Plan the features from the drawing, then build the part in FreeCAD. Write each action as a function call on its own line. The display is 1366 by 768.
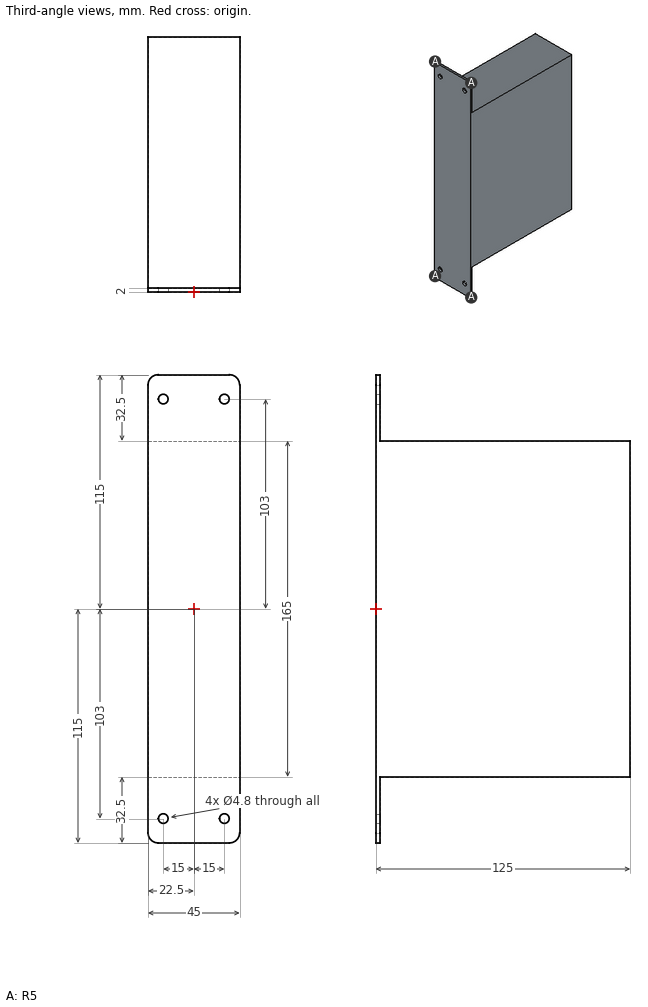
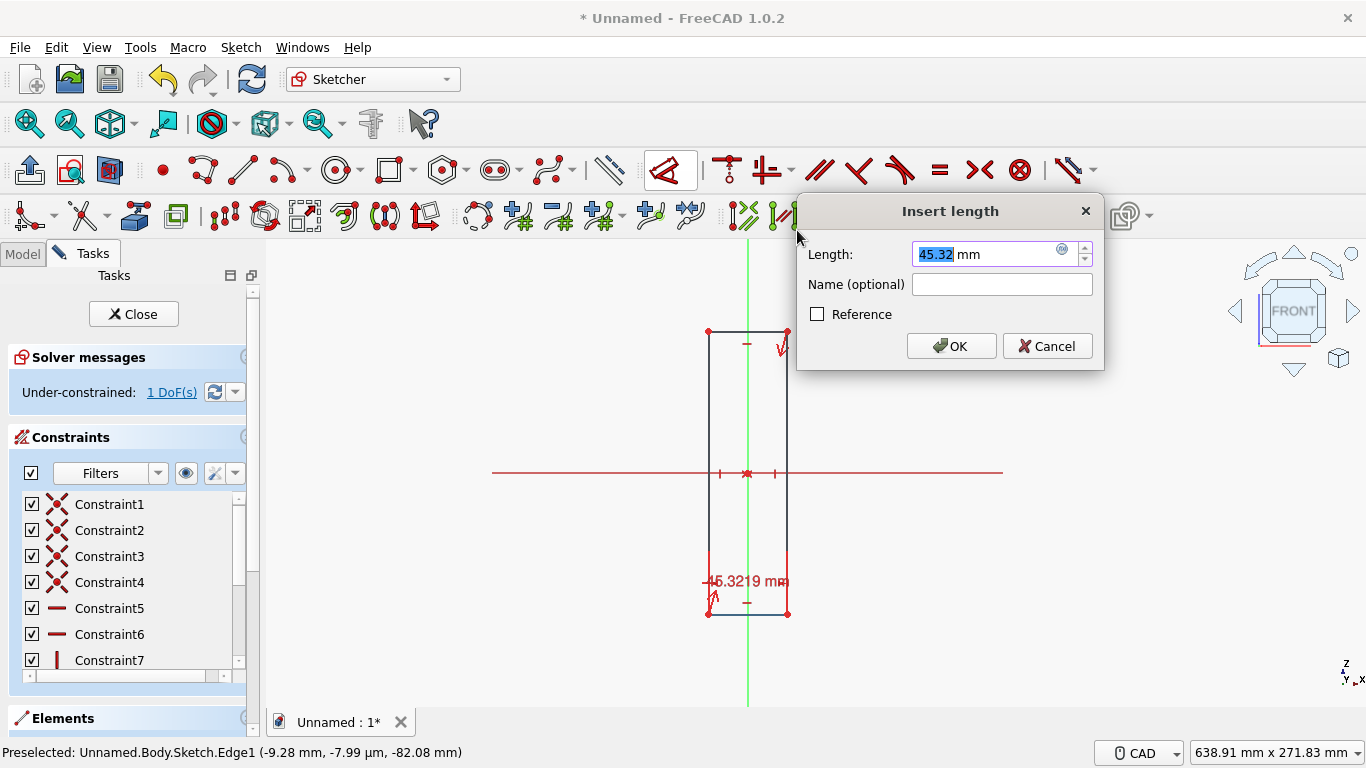
text(45)
key(Return)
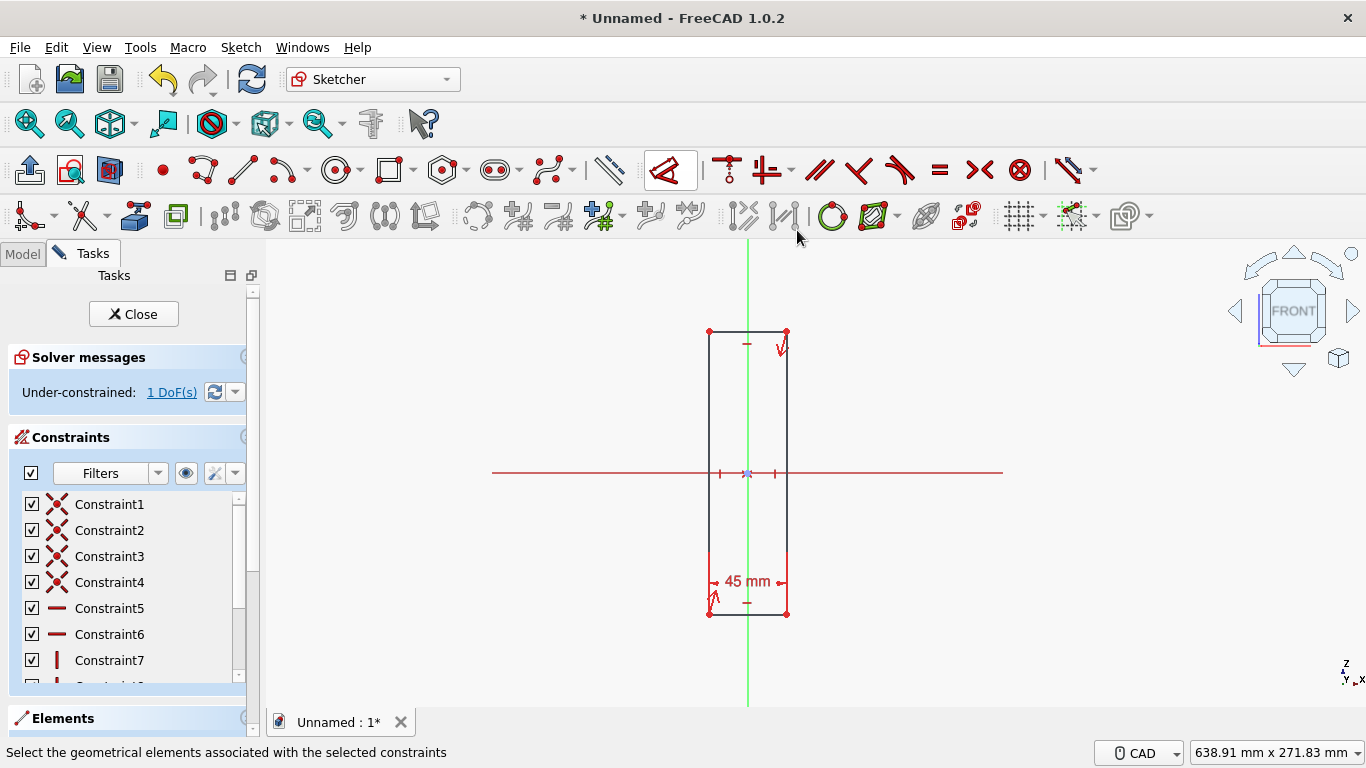
click(787, 530)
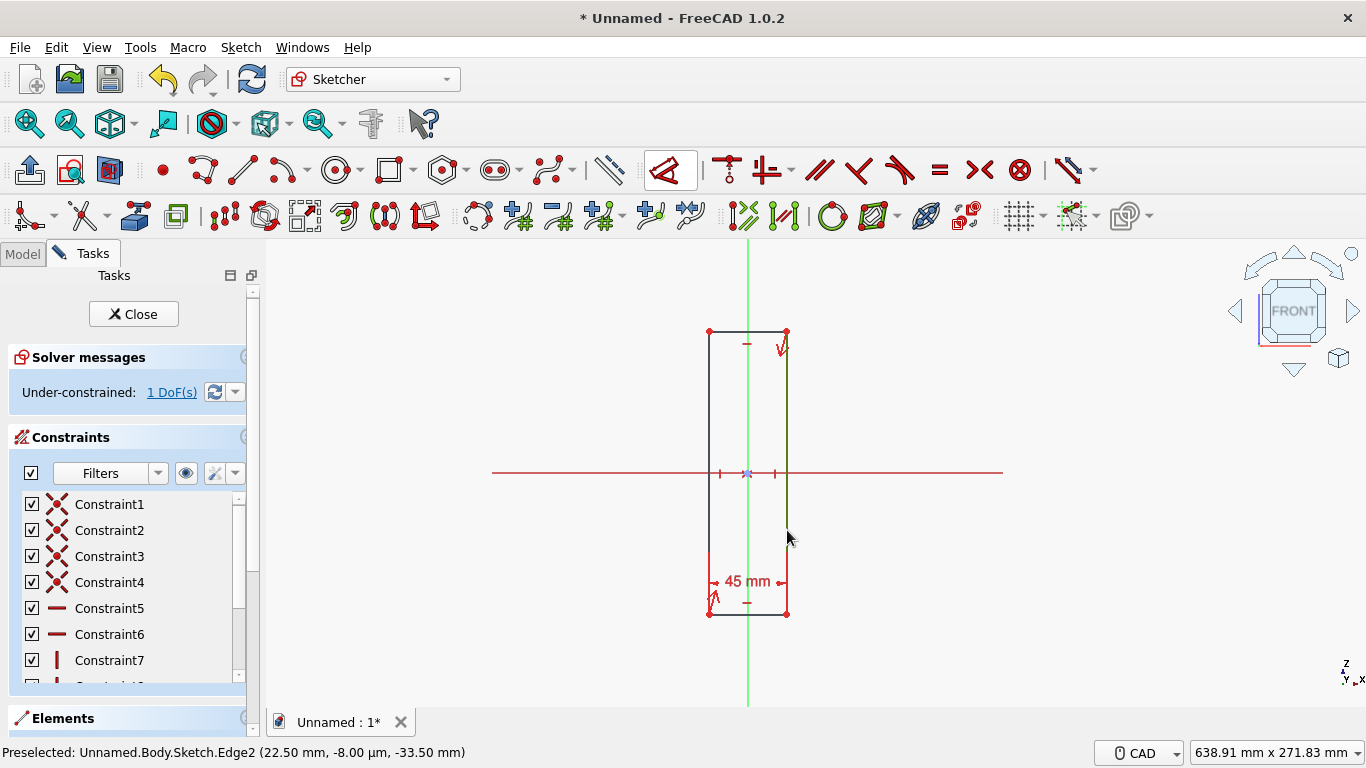
key(i)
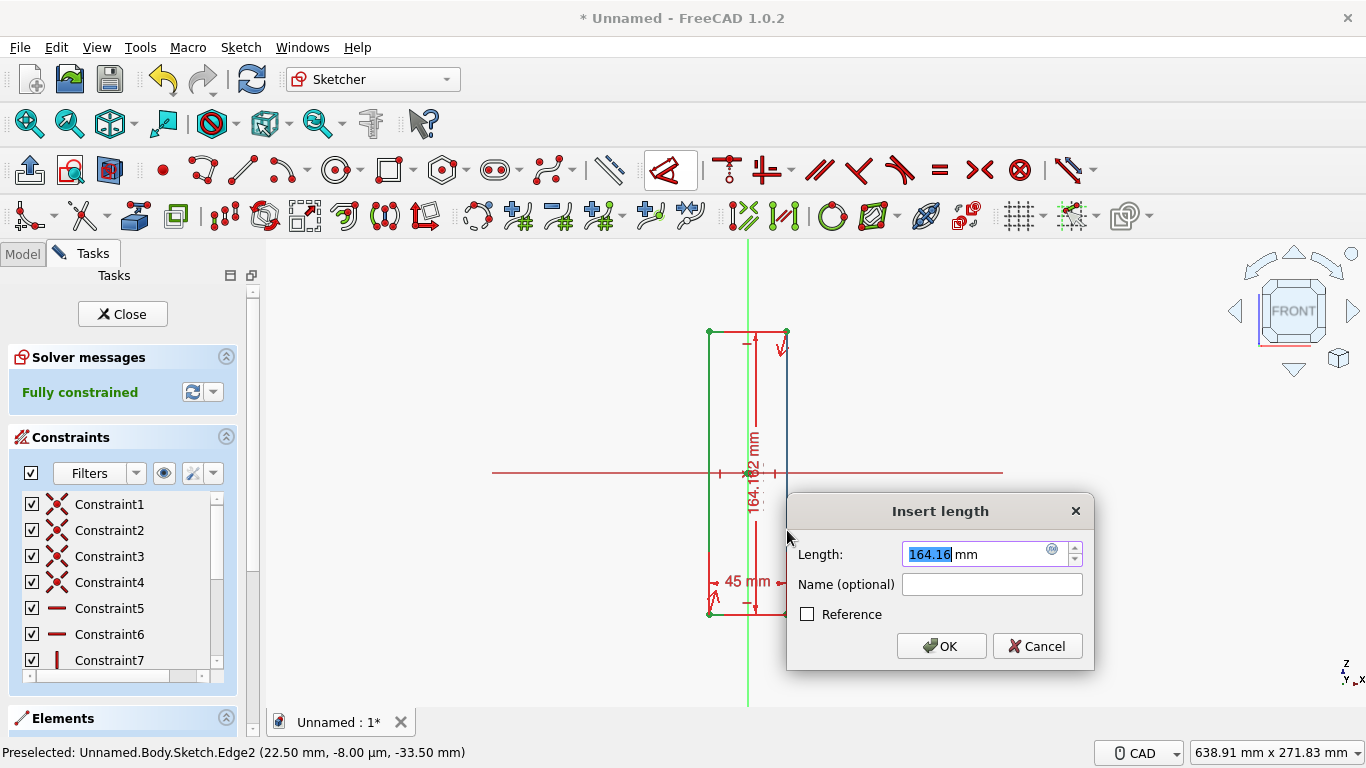
text(165)
key(Return)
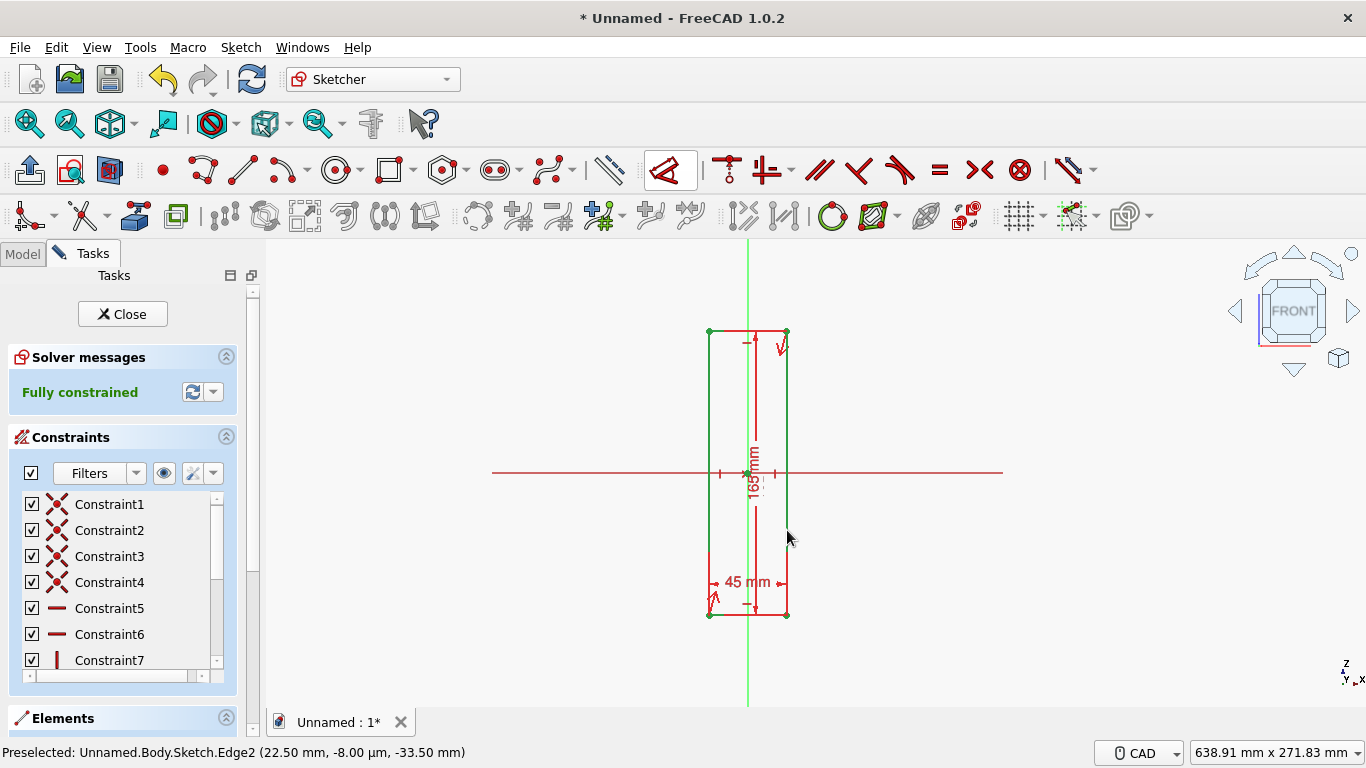
click(123, 314)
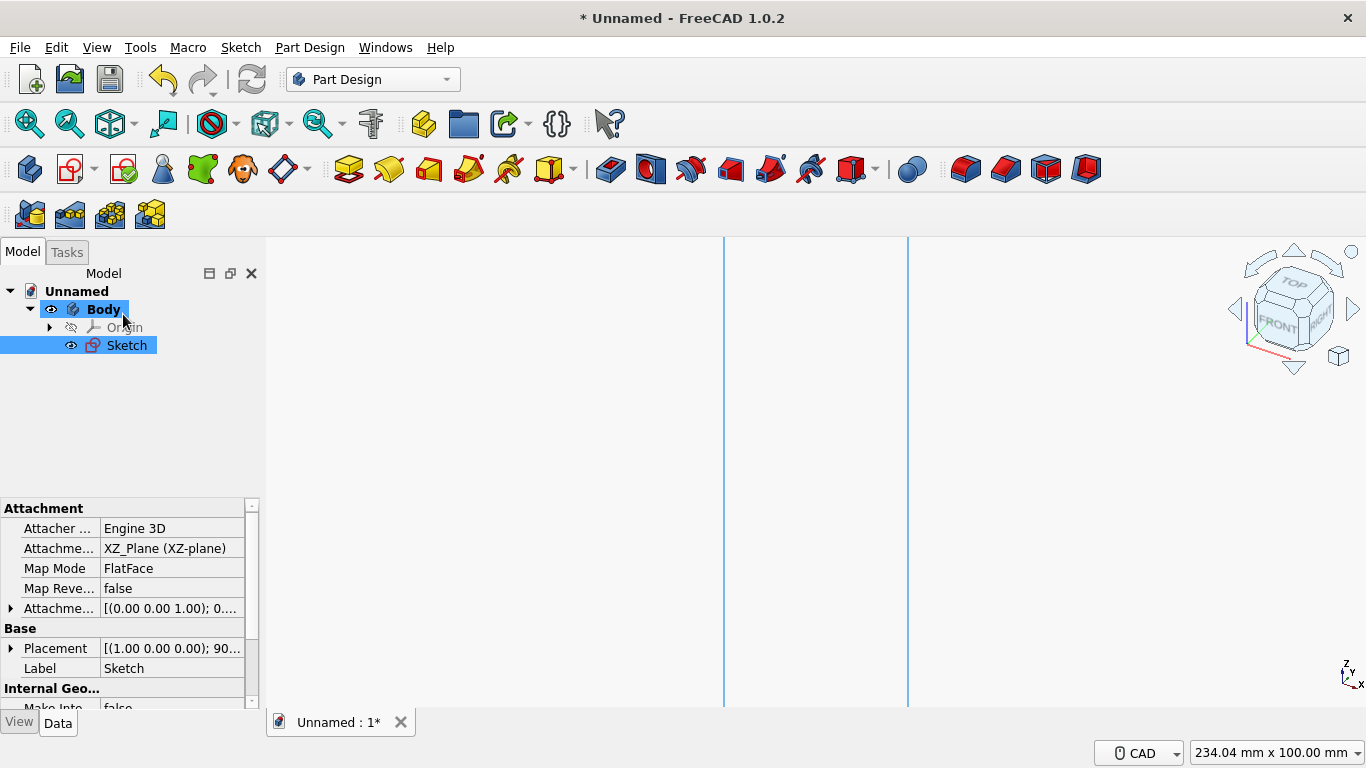
click(350, 170)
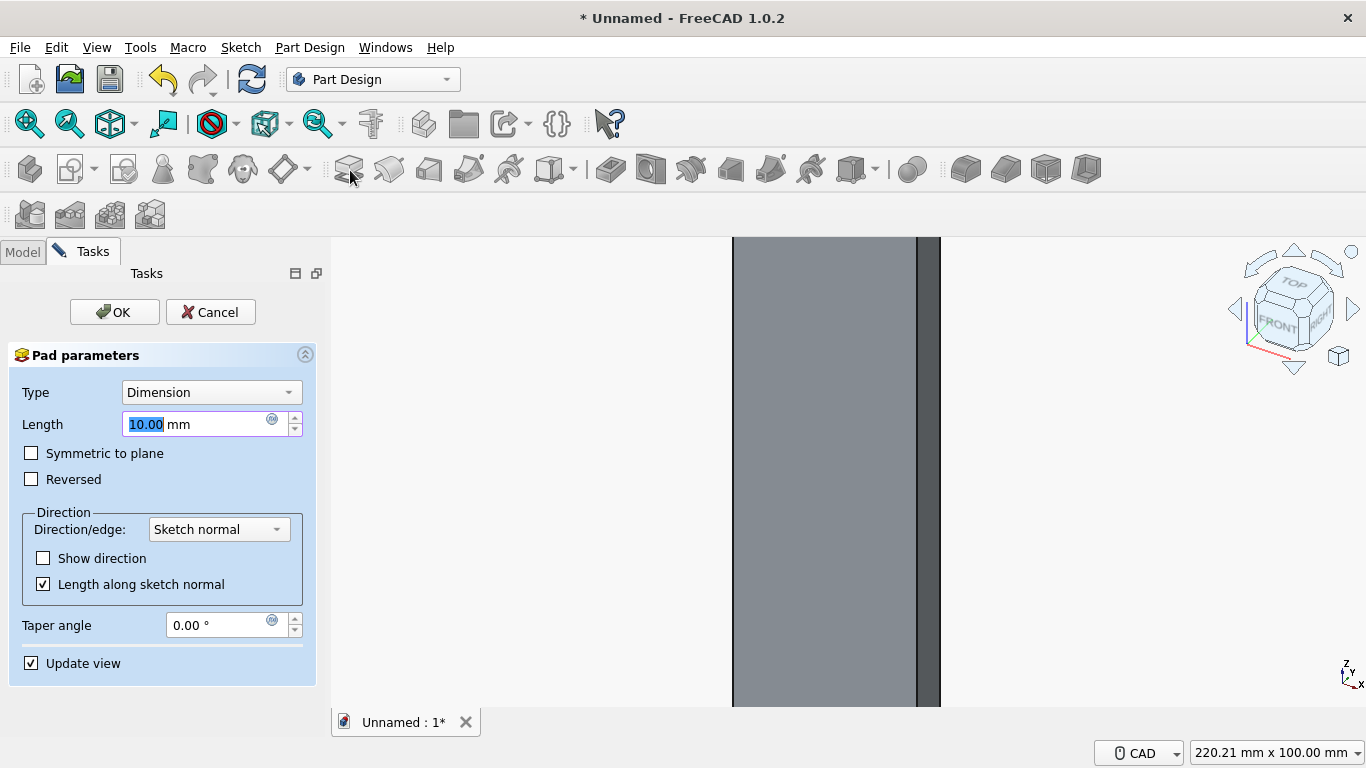
text(125)
key(Tab)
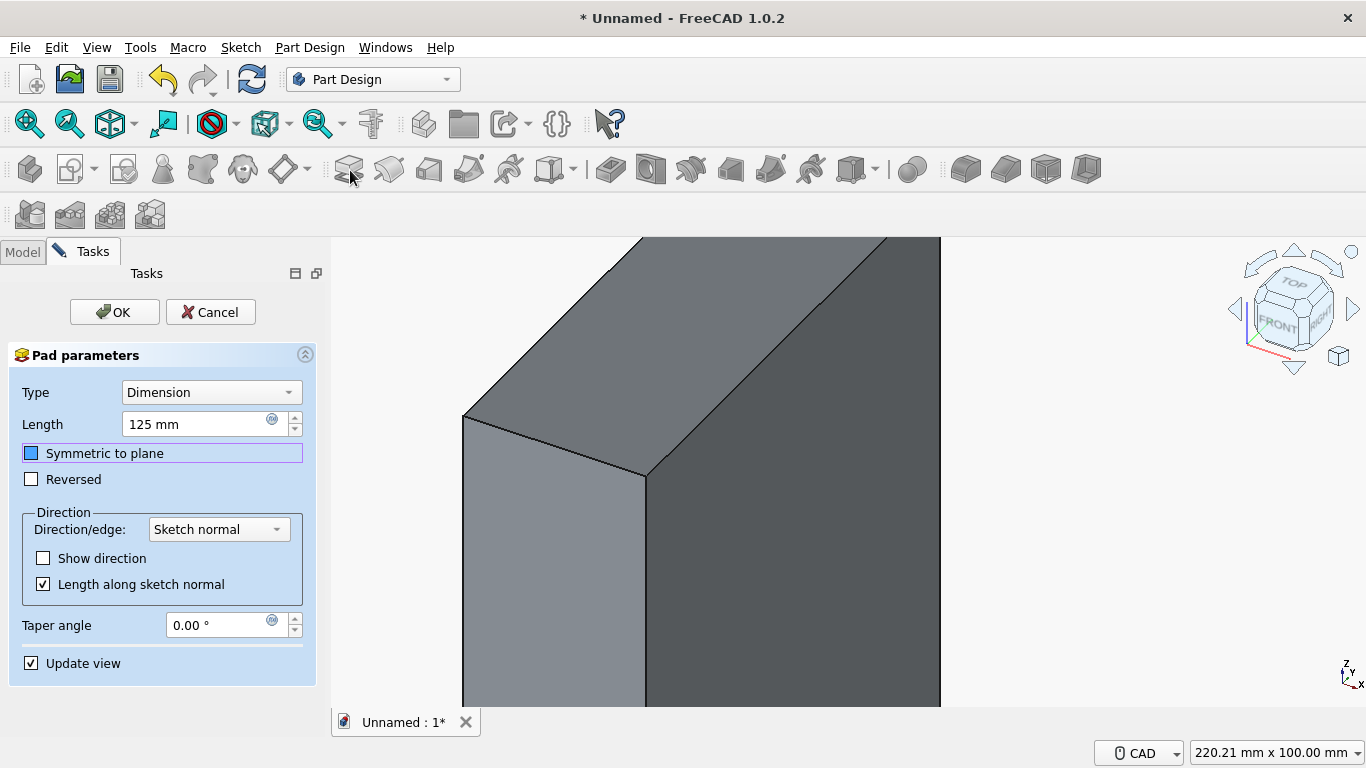
click(30, 479)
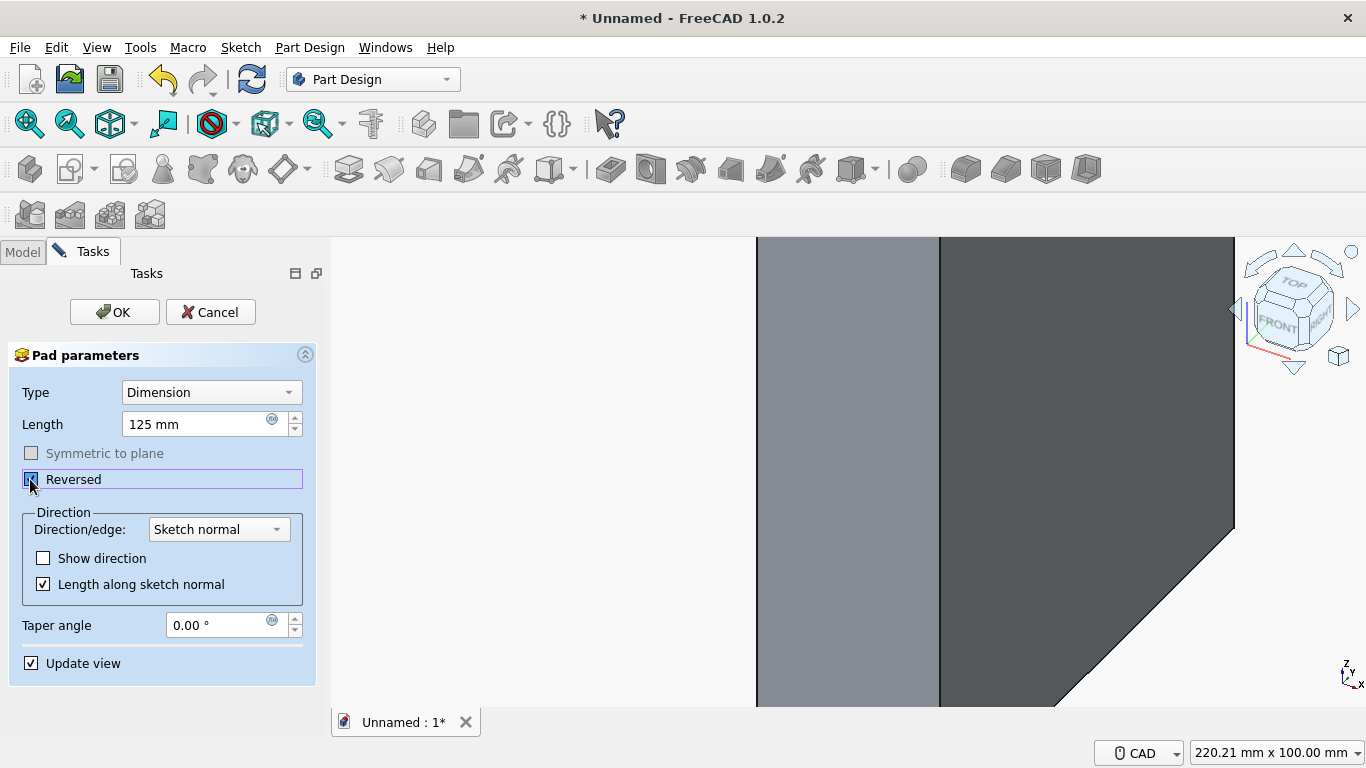
click(115, 312)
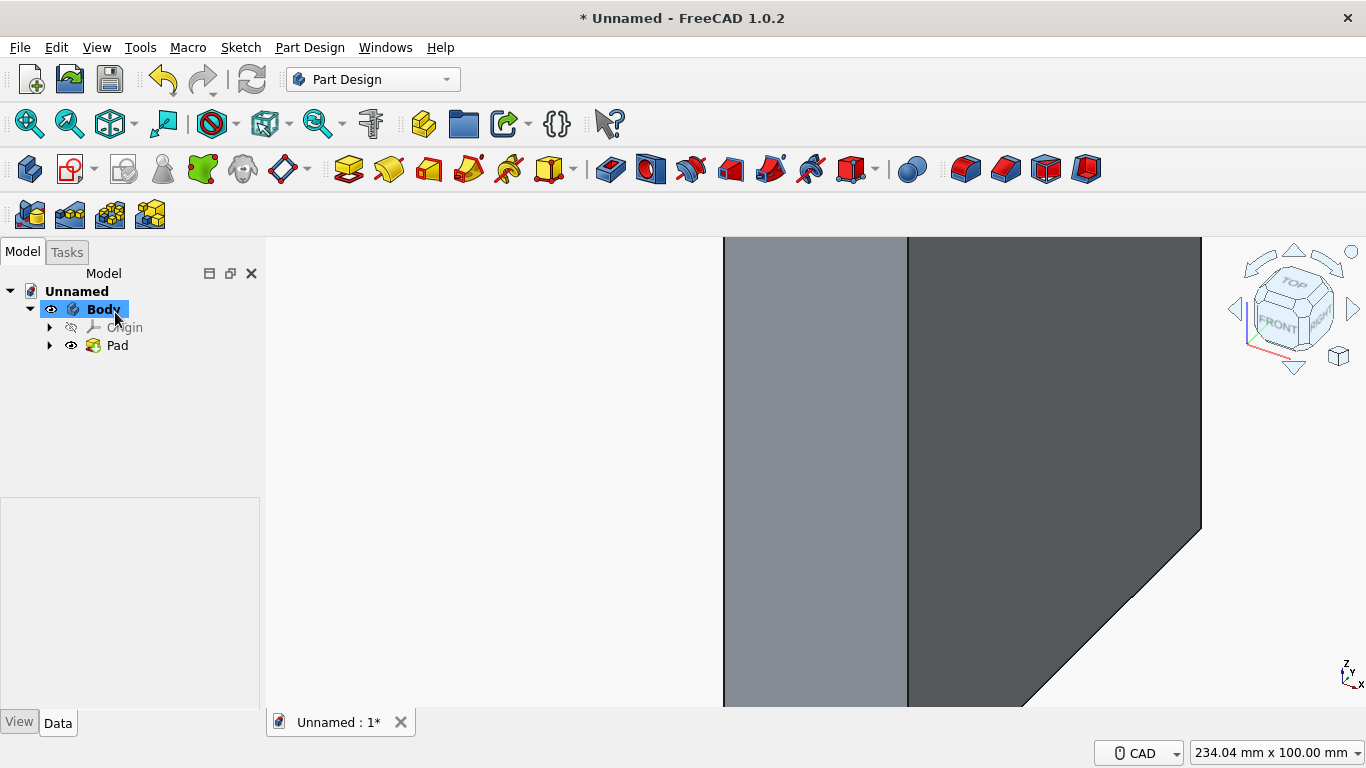
click(30, 124)